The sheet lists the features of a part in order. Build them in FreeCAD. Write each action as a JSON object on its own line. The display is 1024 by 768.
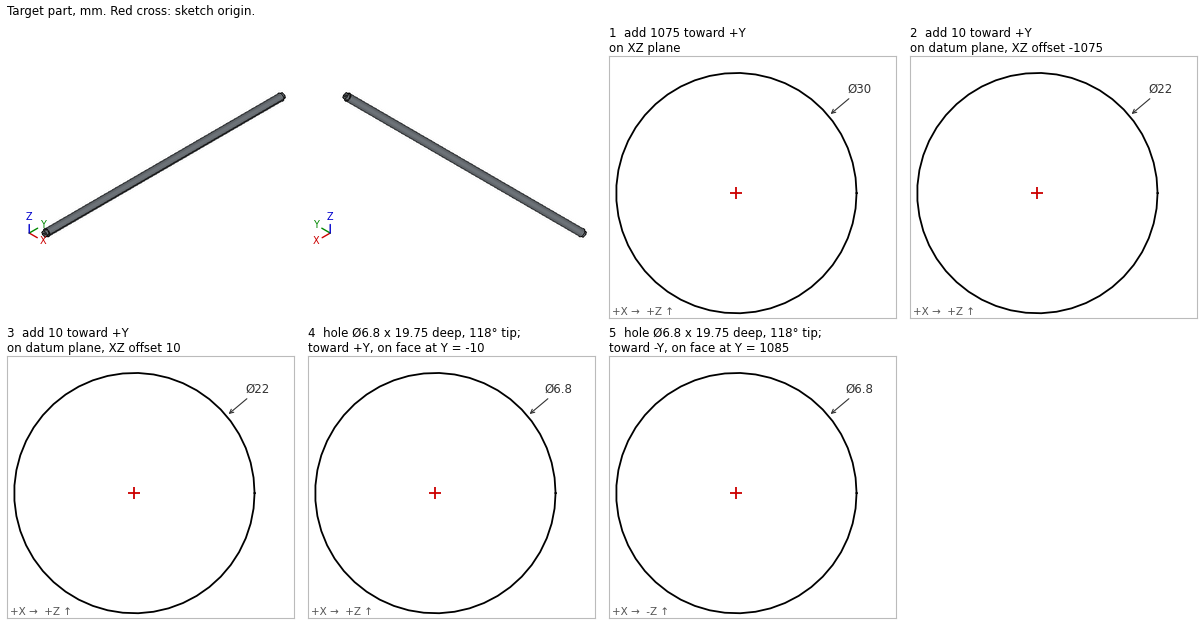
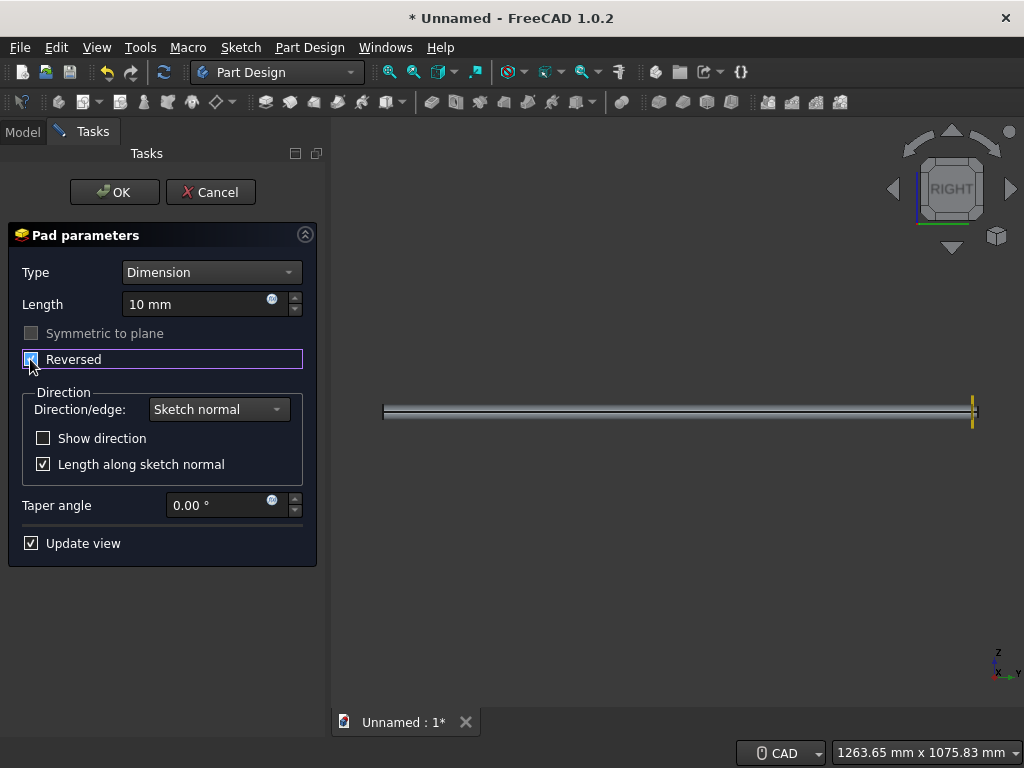
{"action": "left_click", "coordinate": [115, 192]}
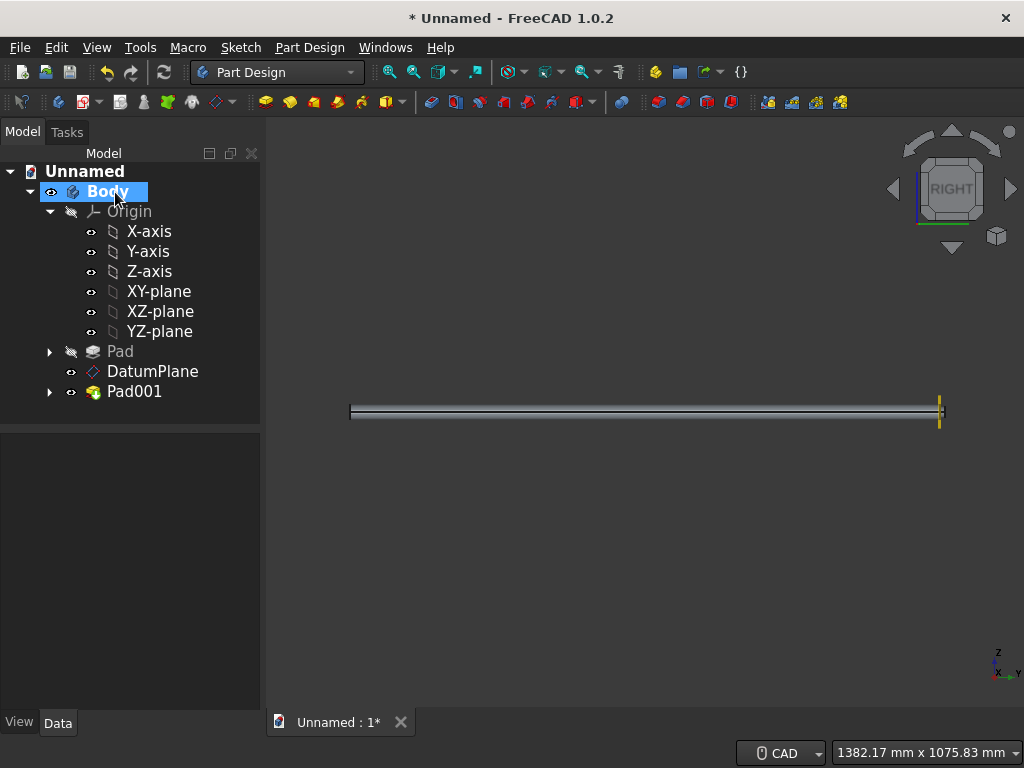
{"action": "left_click", "coordinate": [116, 372]}
{"action": "key", "text": "space"}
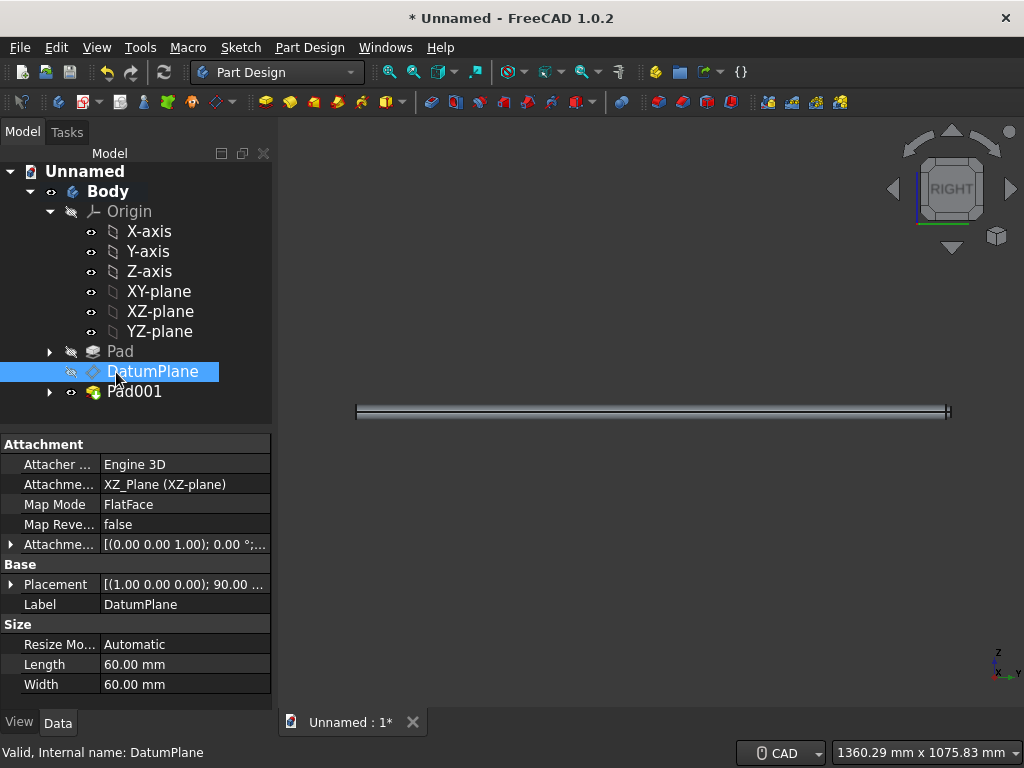
{"action": "left_click", "coordinate": [136, 312]}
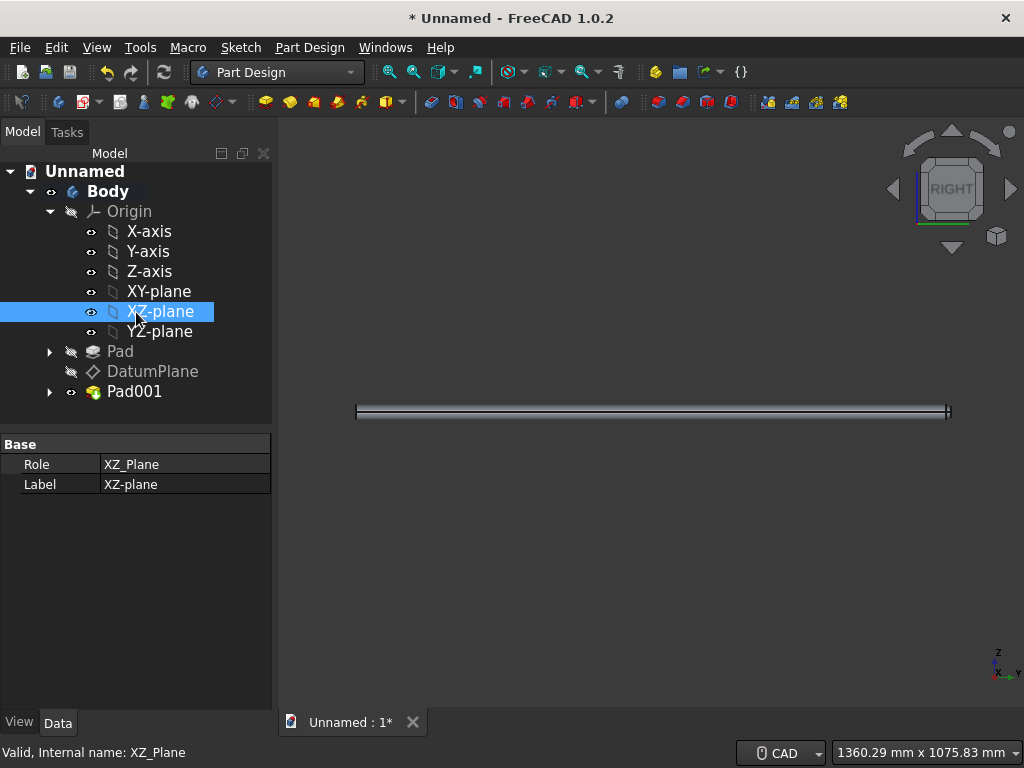
{"action": "left_click", "coordinate": [216, 102]}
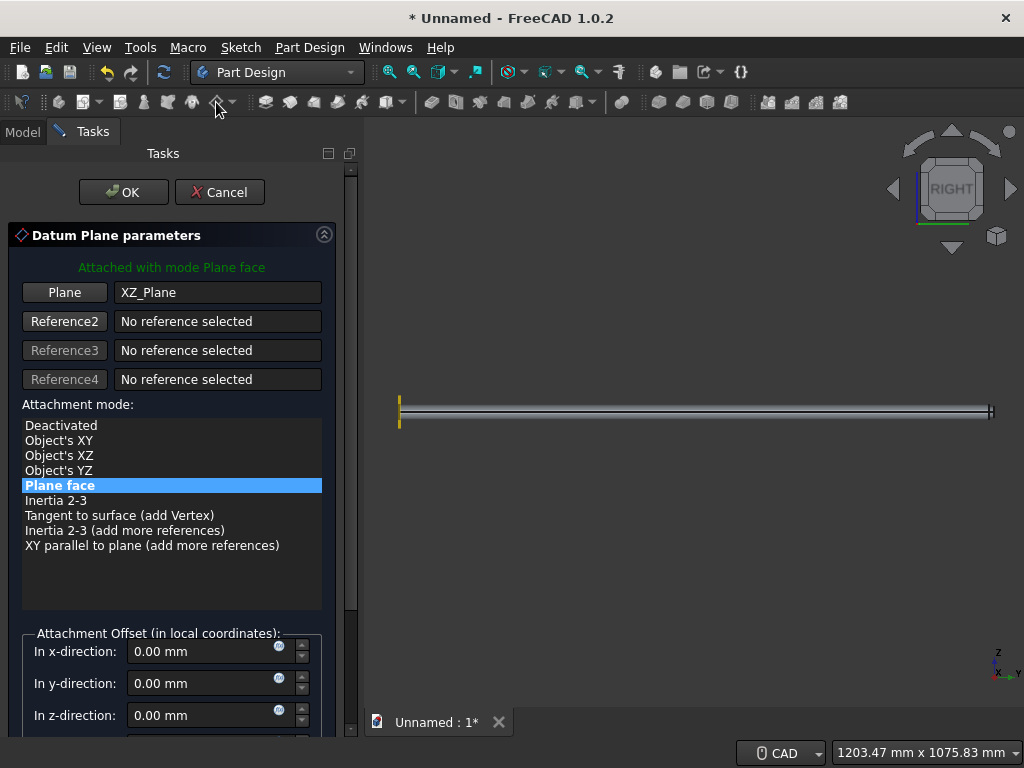
{"action": "triple_click", "coordinate": [210, 715]}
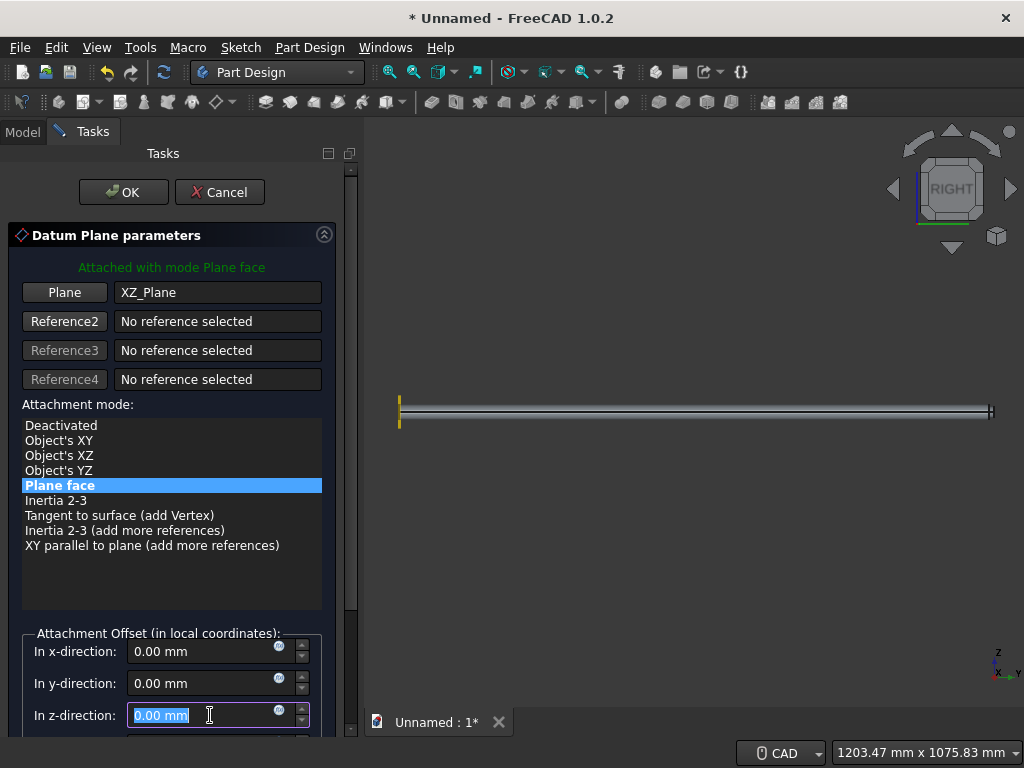
{"action": "type", "text": "10"}
{"action": "key", "text": "Tab"}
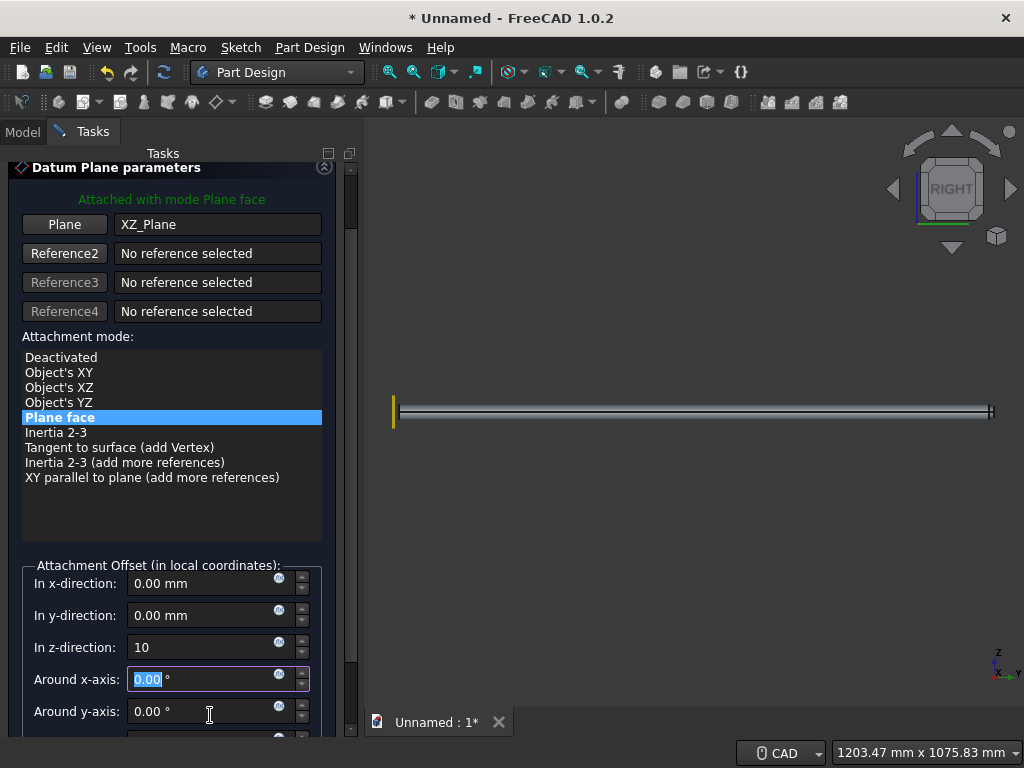
{"action": "scroll", "coordinate": [351, 450], "scroll_direction": "up", "scroll_amount": 2}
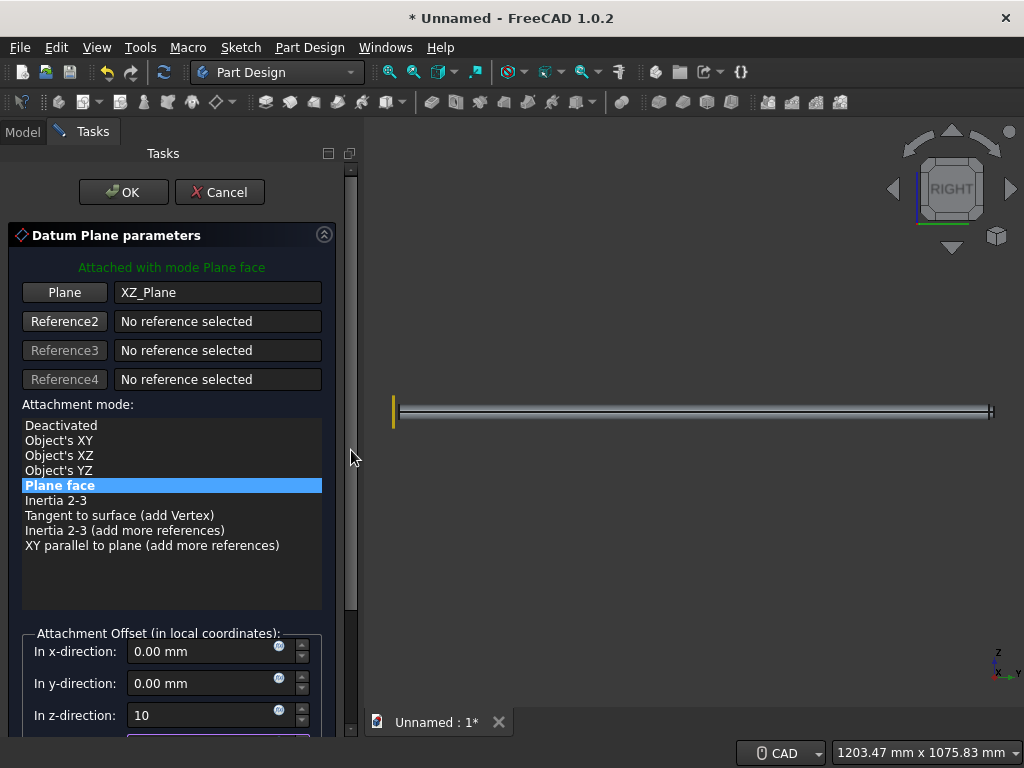
{"action": "left_click", "coordinate": [124, 192]}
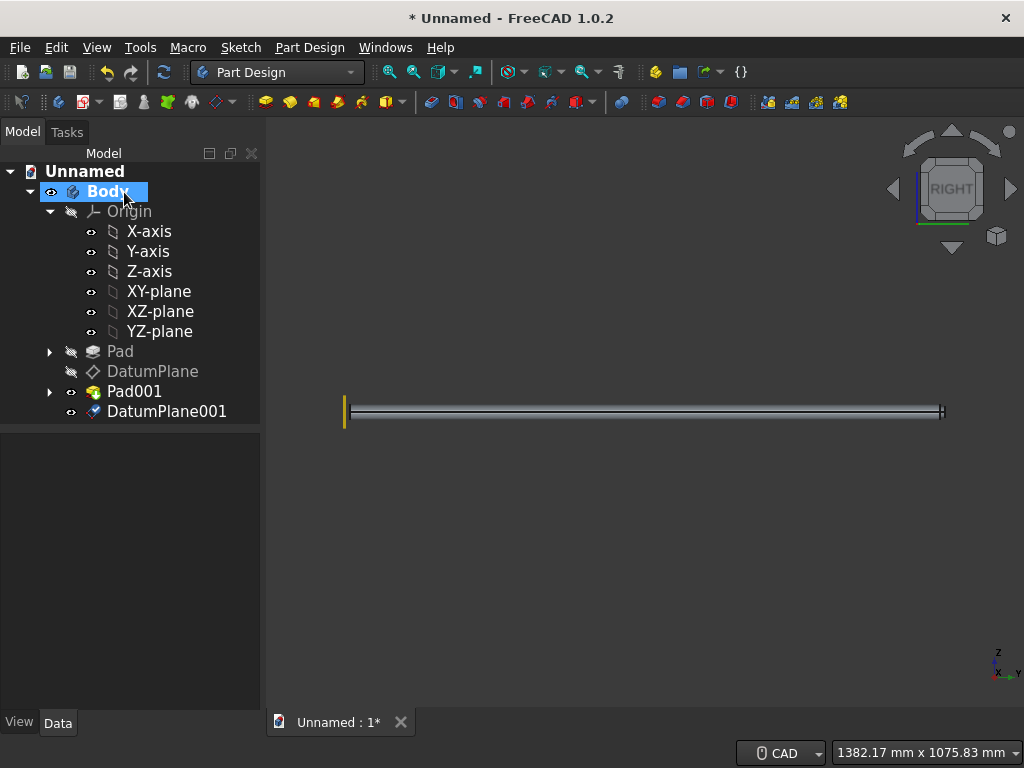
{"action": "left_click", "coordinate": [116, 412]}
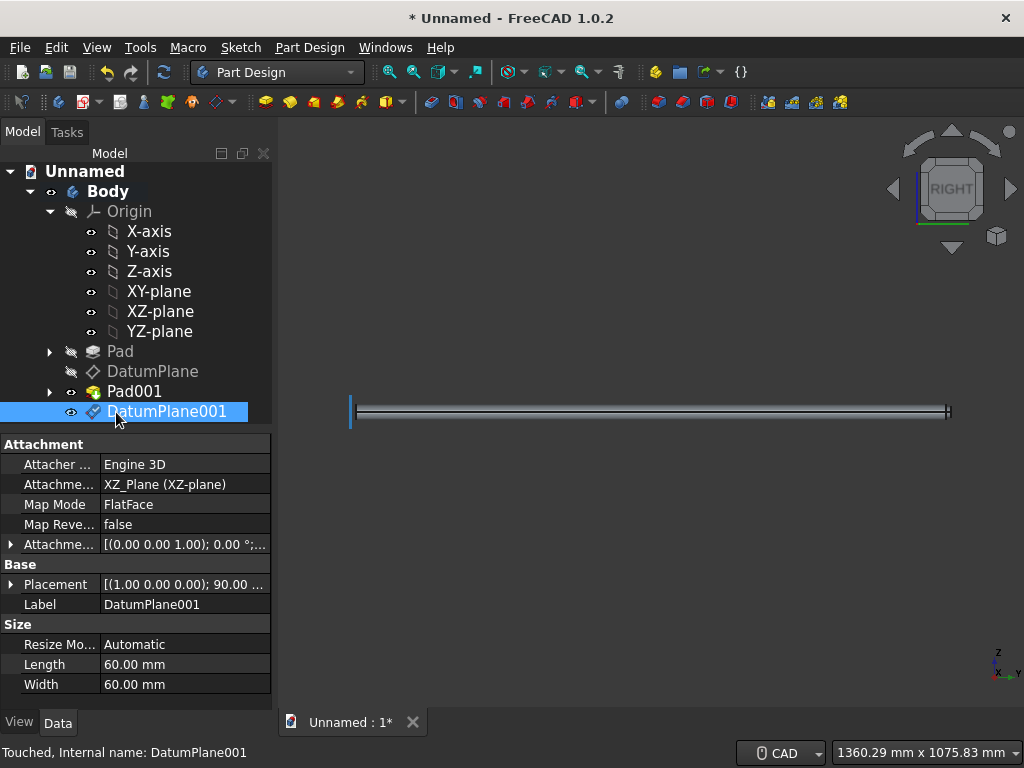
{"action": "left_click", "coordinate": [84, 102]}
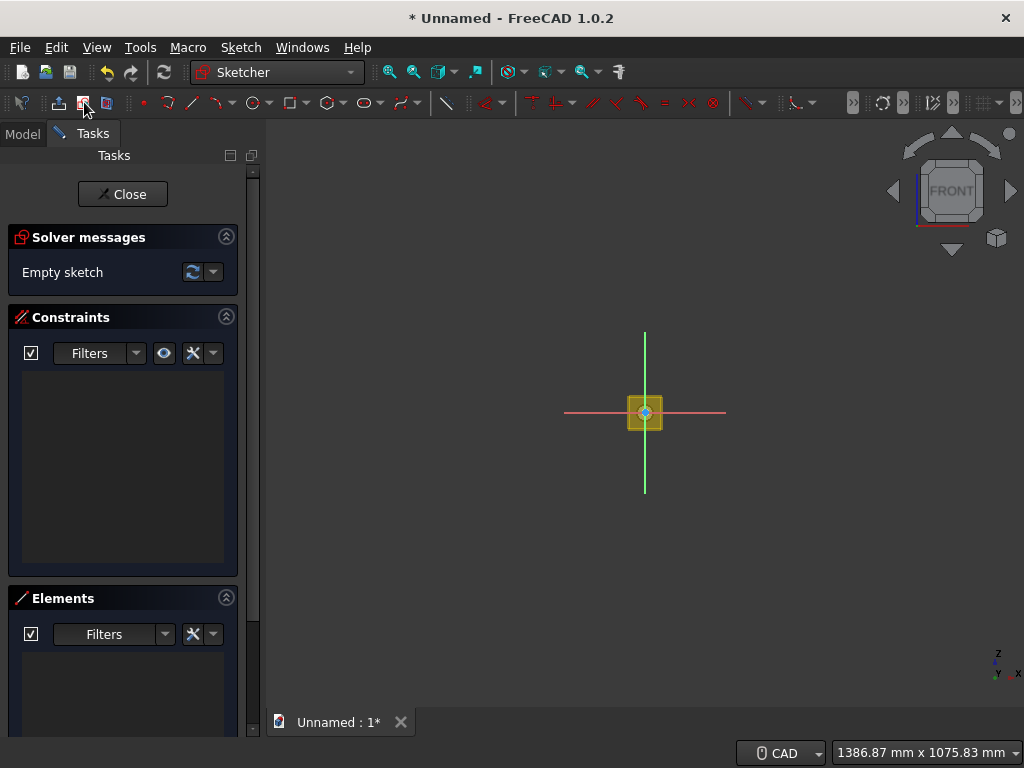
{"action": "scroll", "coordinate": [649, 413], "scroll_direction": "up", "scroll_amount": 15}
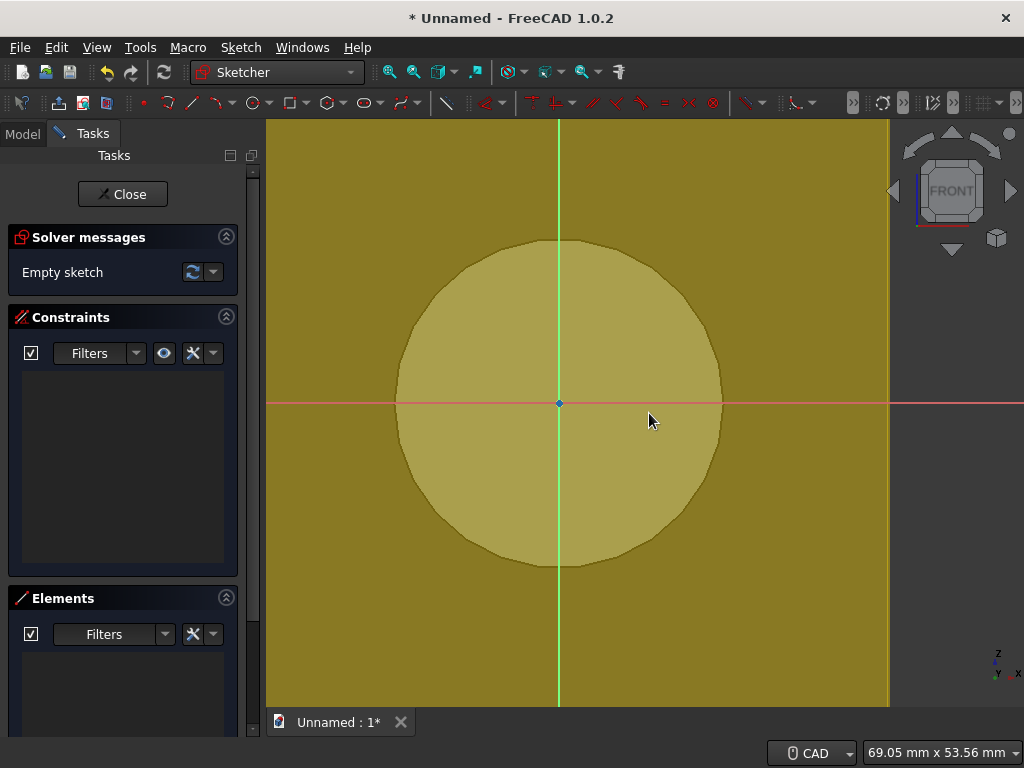
{"action": "scroll", "coordinate": [523, 384], "scroll_direction": "up", "scroll_amount": 2}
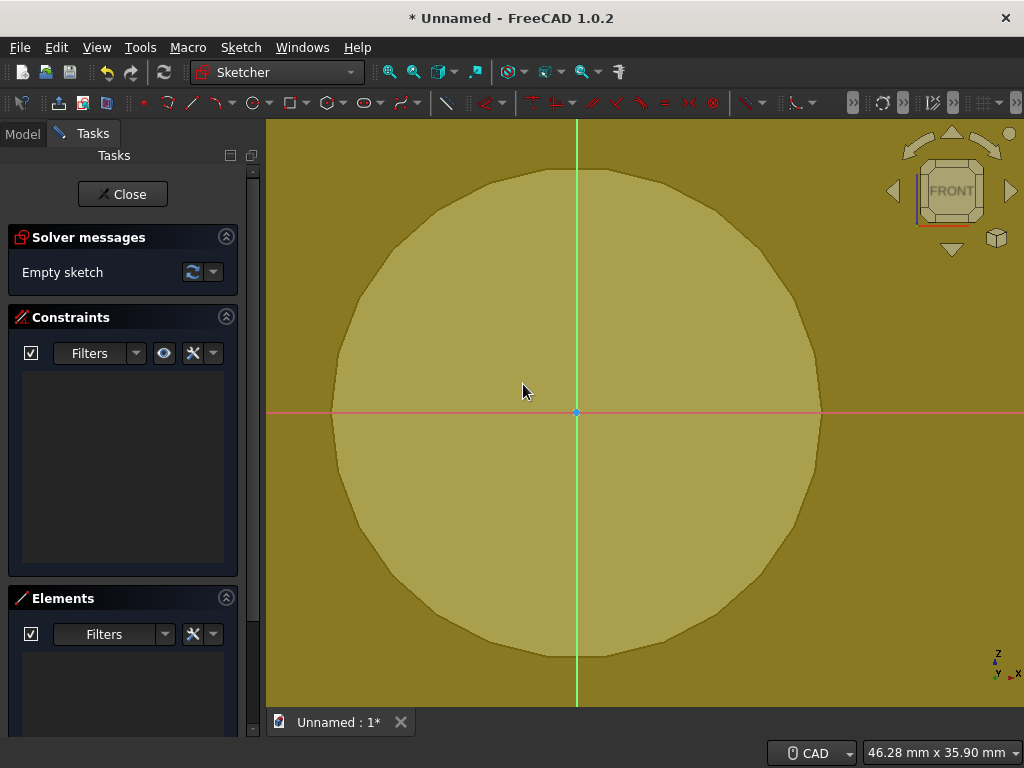
{"action": "left_click", "coordinate": [254, 104]}